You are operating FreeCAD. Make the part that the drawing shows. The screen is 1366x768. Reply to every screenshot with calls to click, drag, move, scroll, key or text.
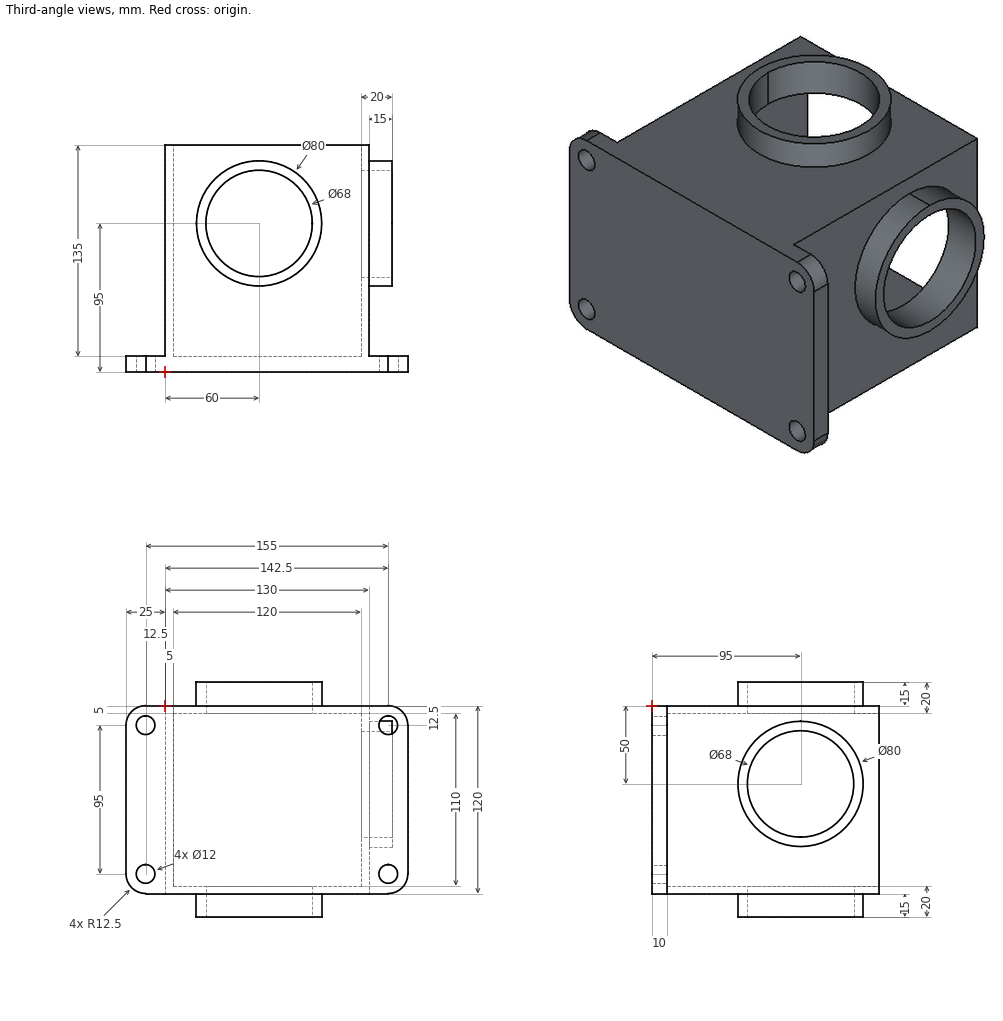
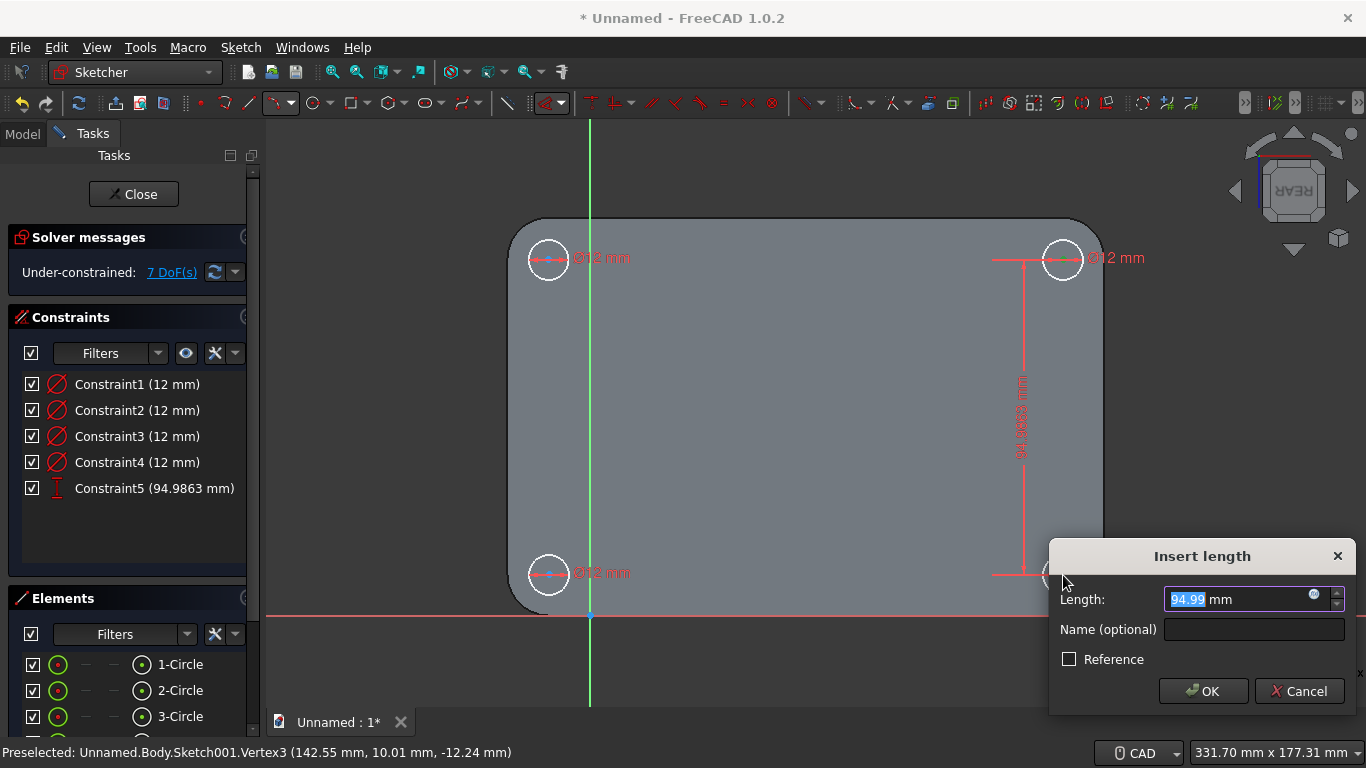
text(95)
key(Return)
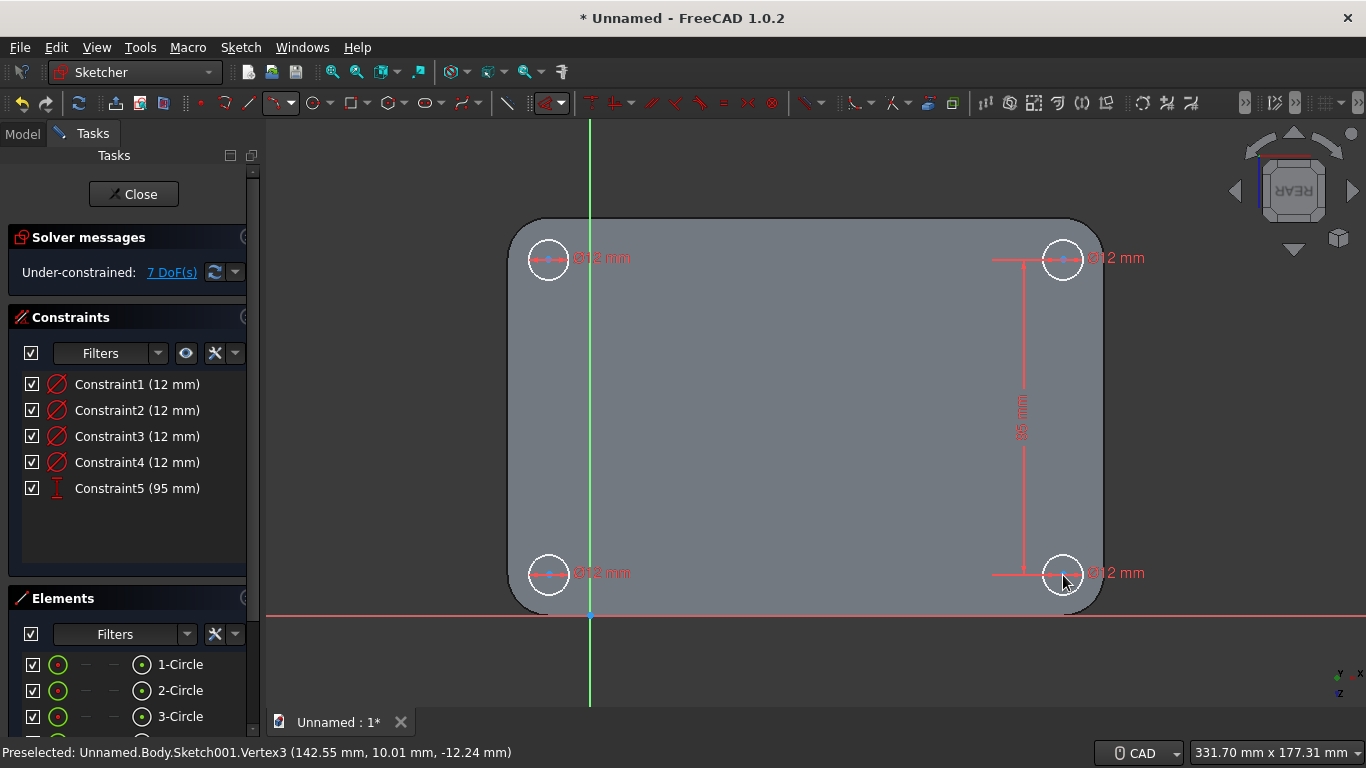
click(549, 260)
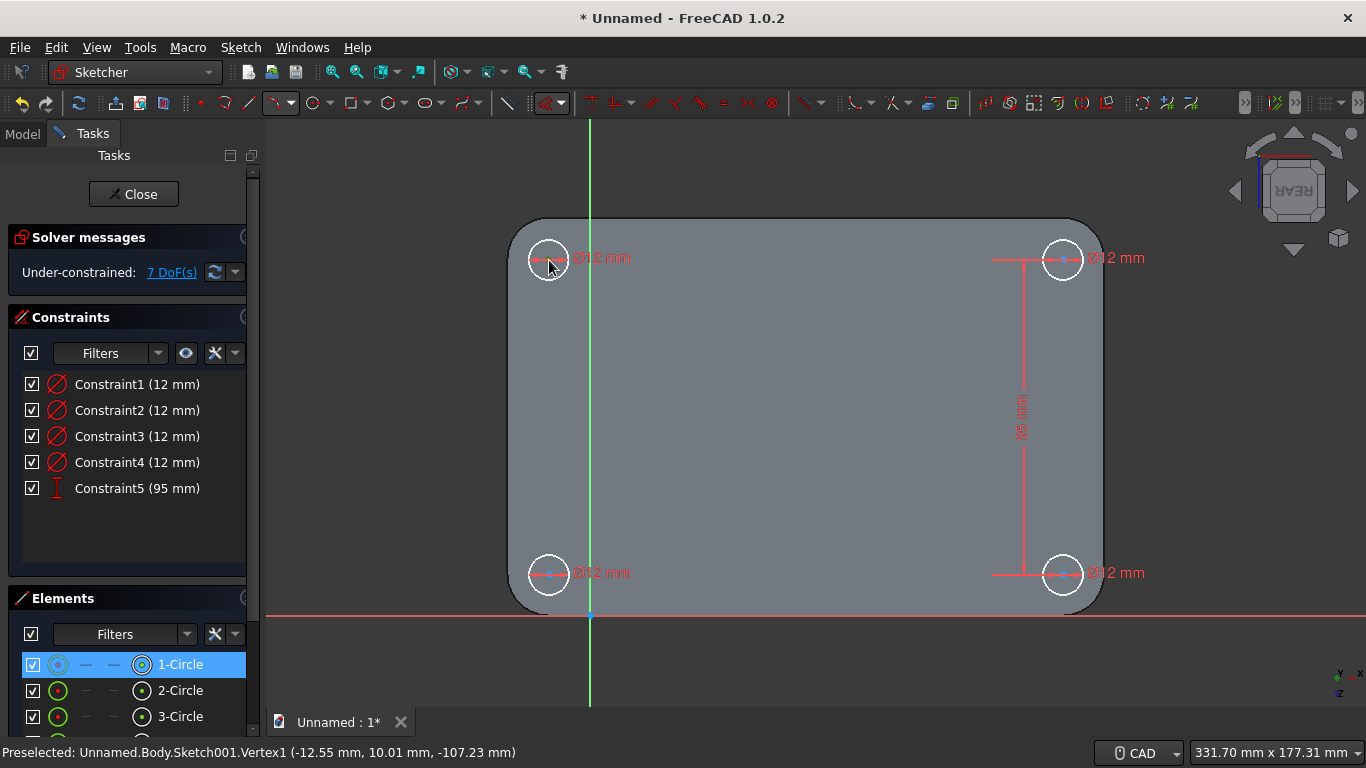
click(1063, 575)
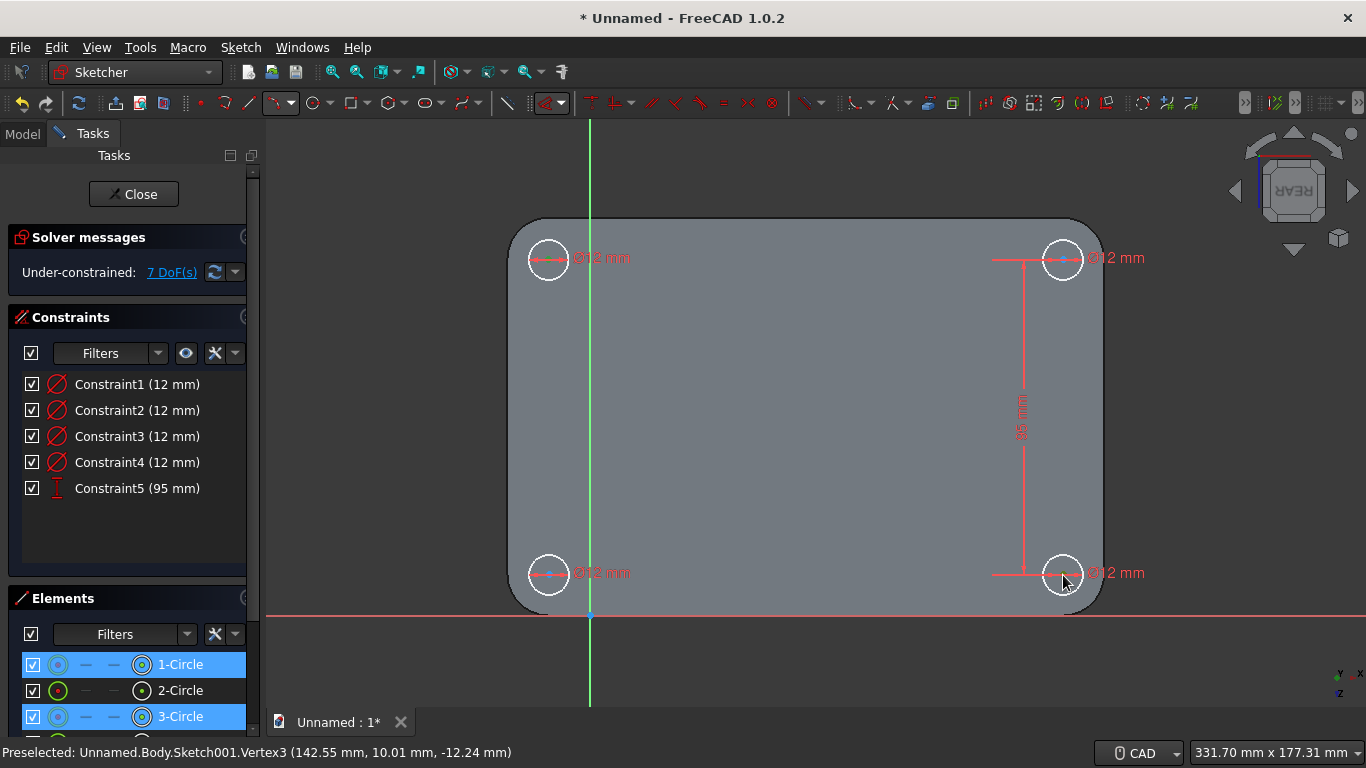
click(564, 104)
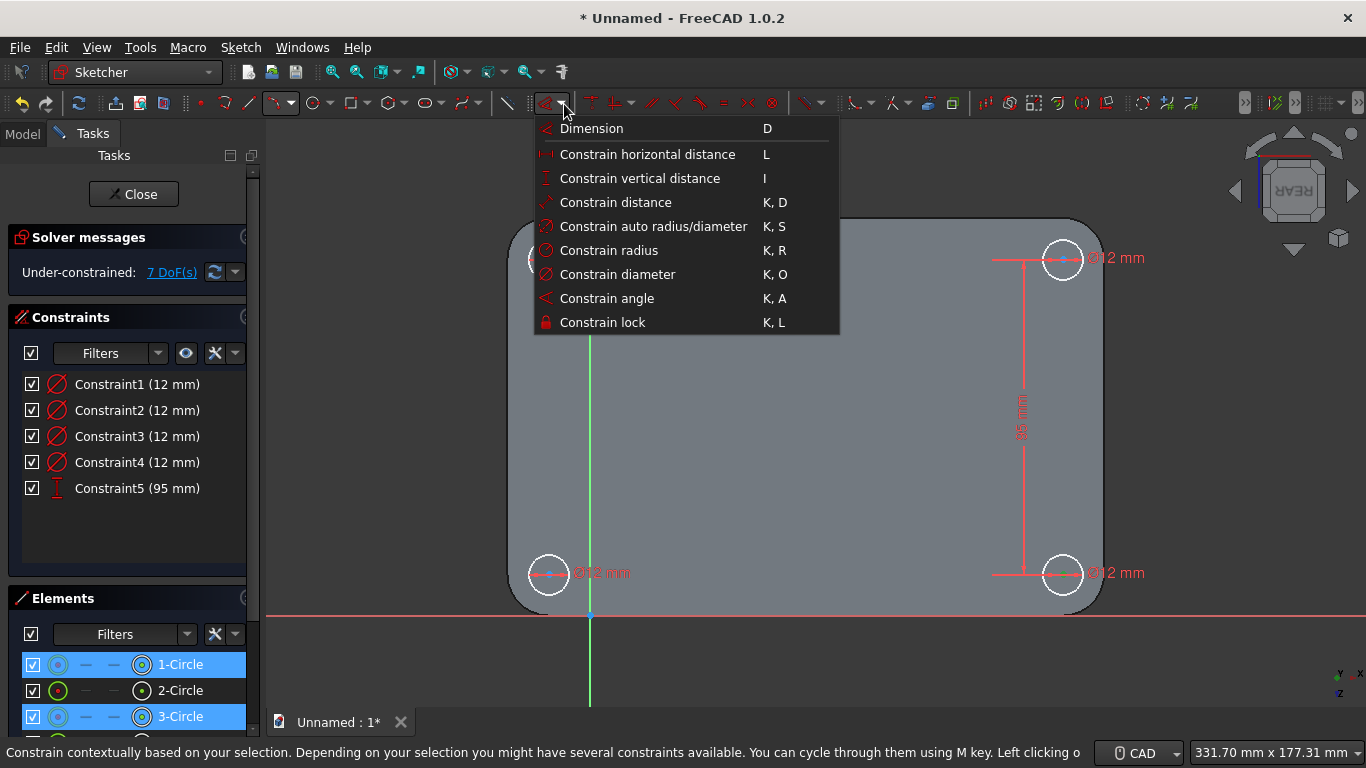
click(687, 178)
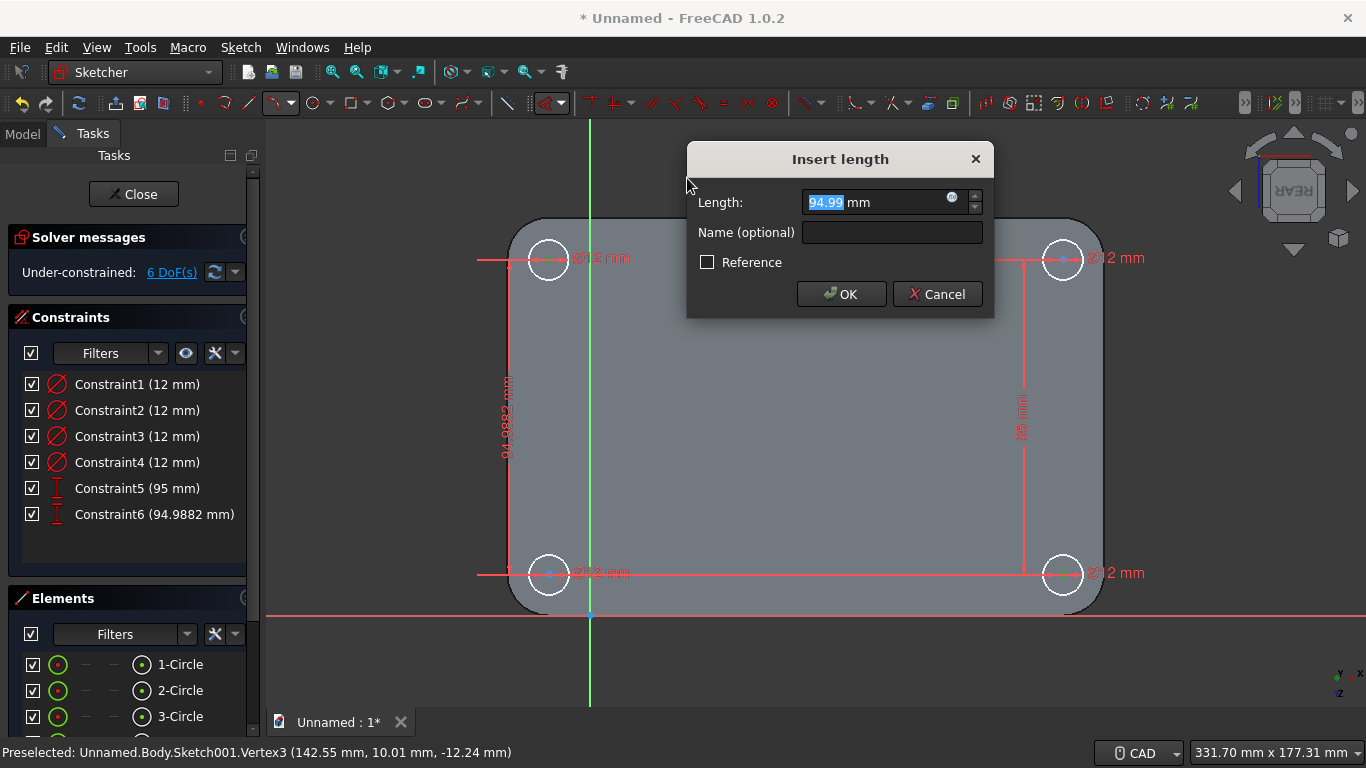
text(95)
key(Return)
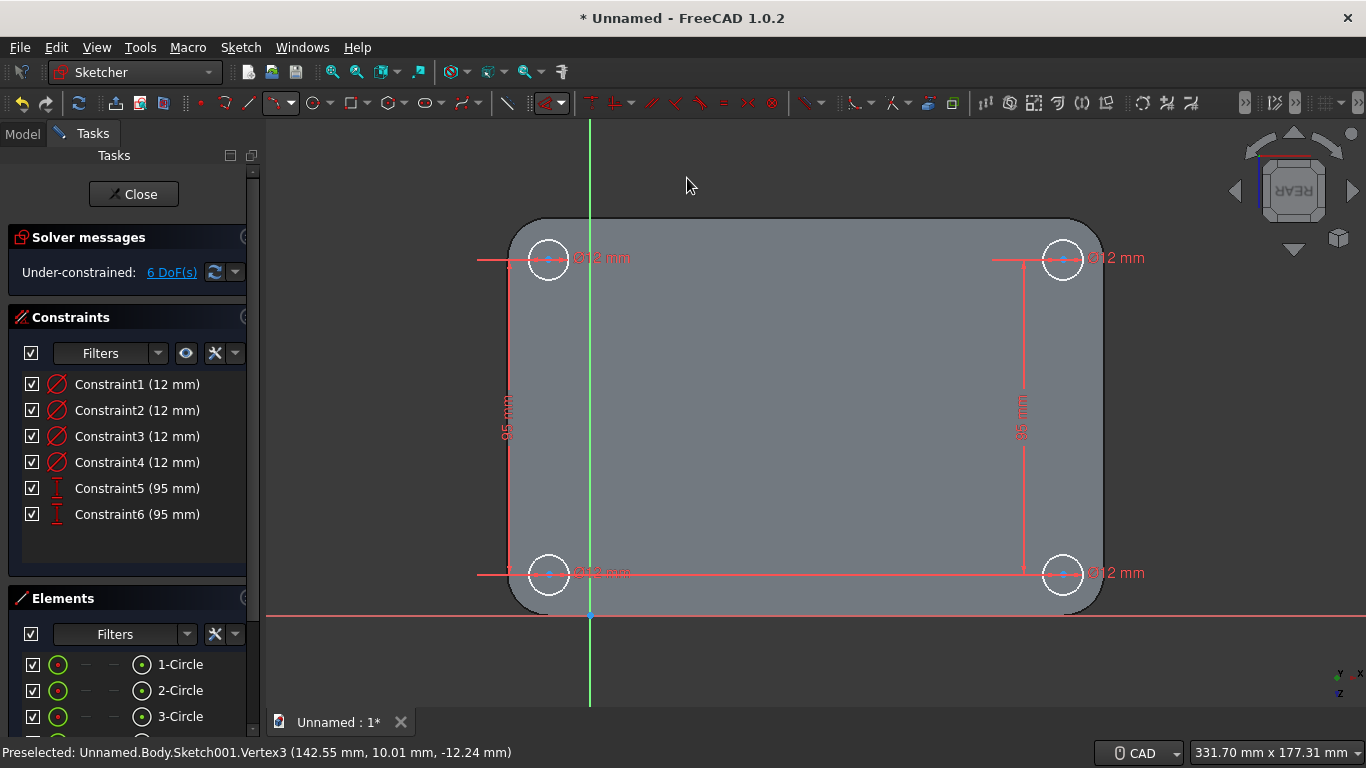
click(549, 260)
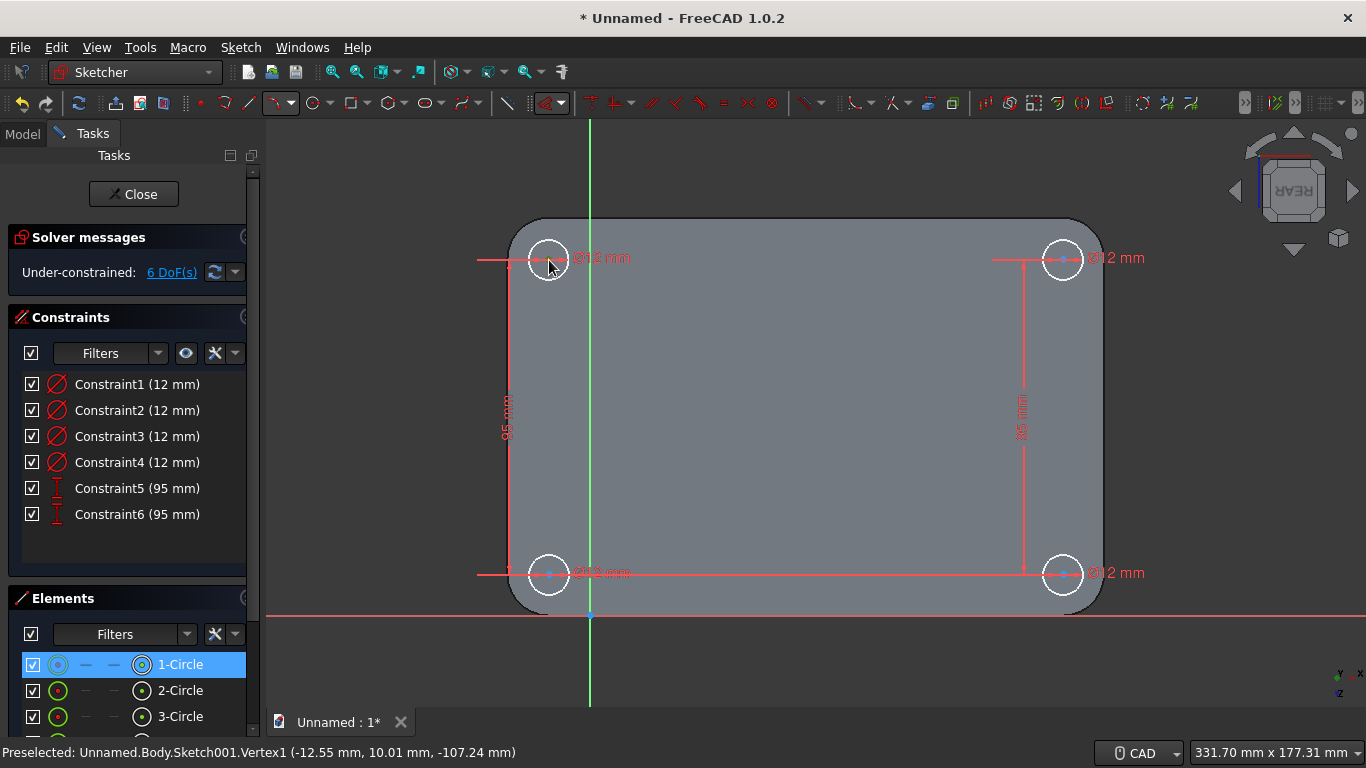
click(549, 575)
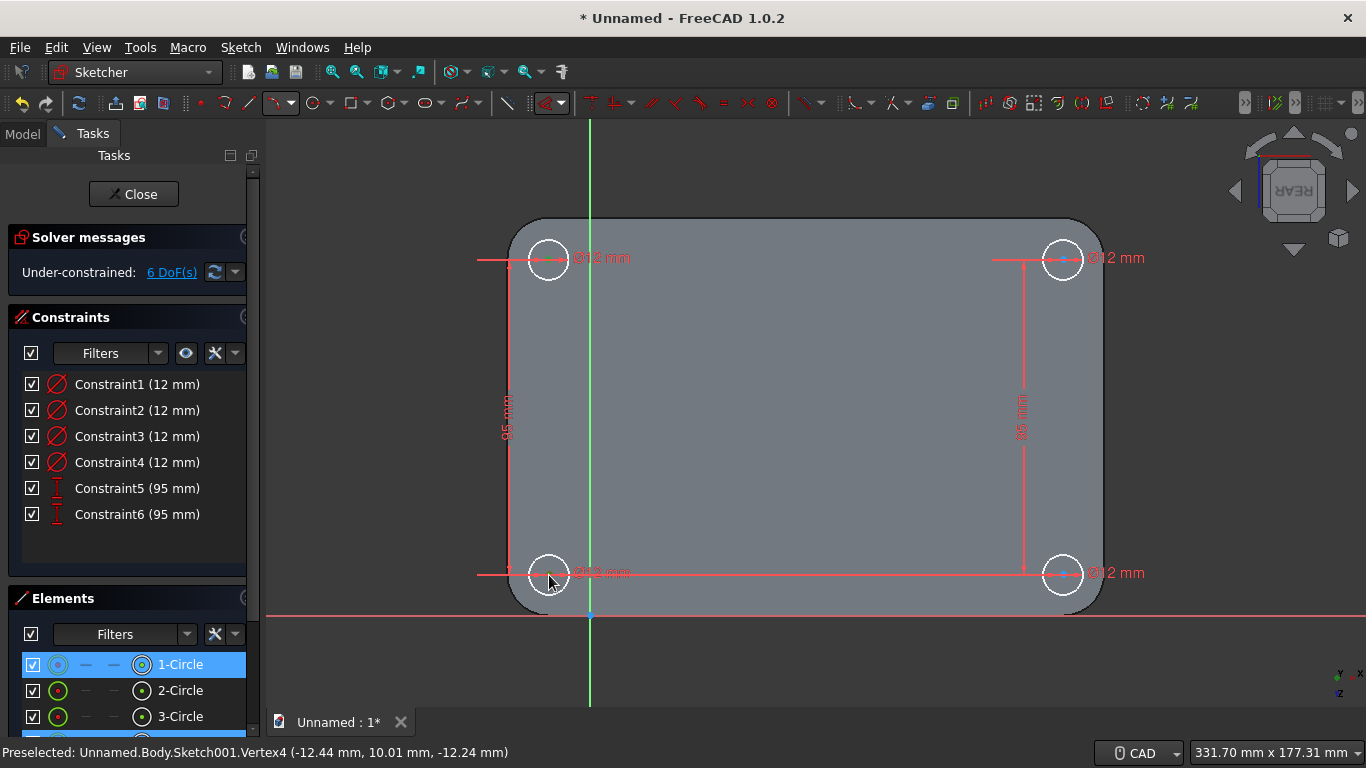
key(i)